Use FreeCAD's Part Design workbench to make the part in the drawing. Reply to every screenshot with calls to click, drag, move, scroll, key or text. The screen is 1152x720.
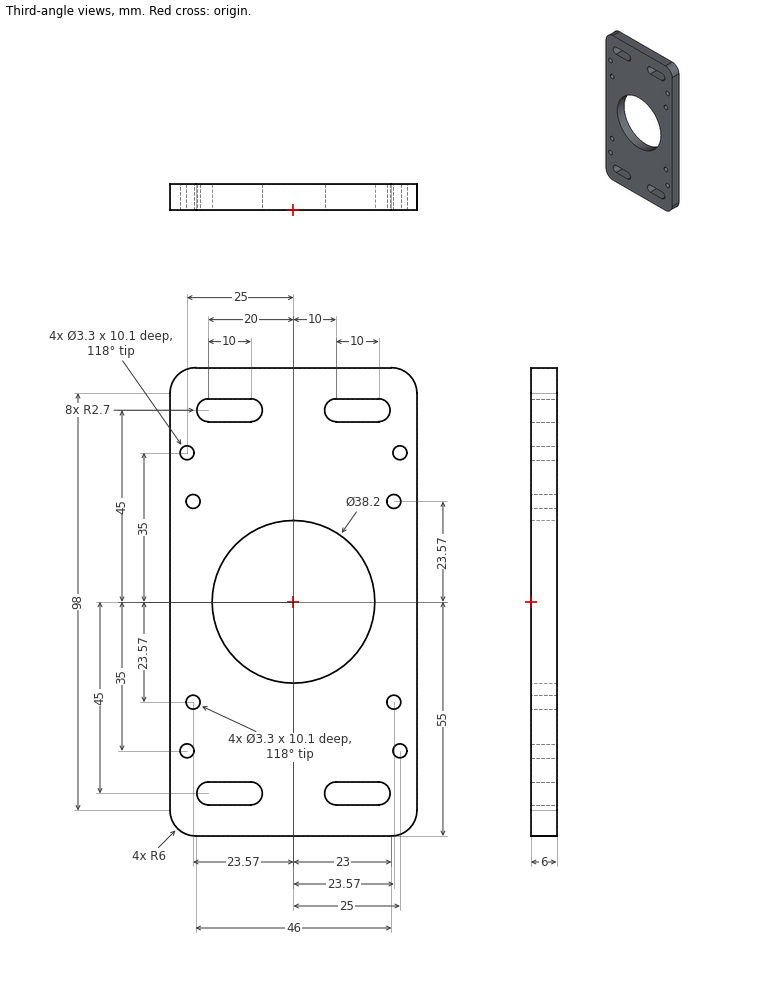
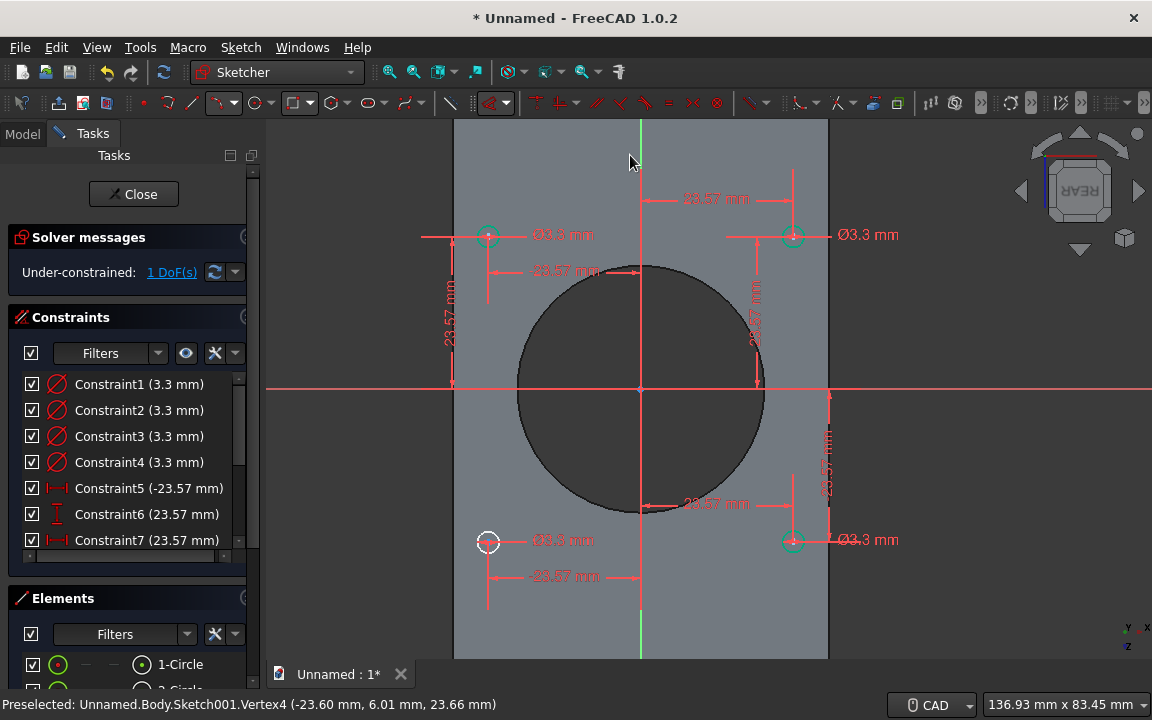
click(488, 542)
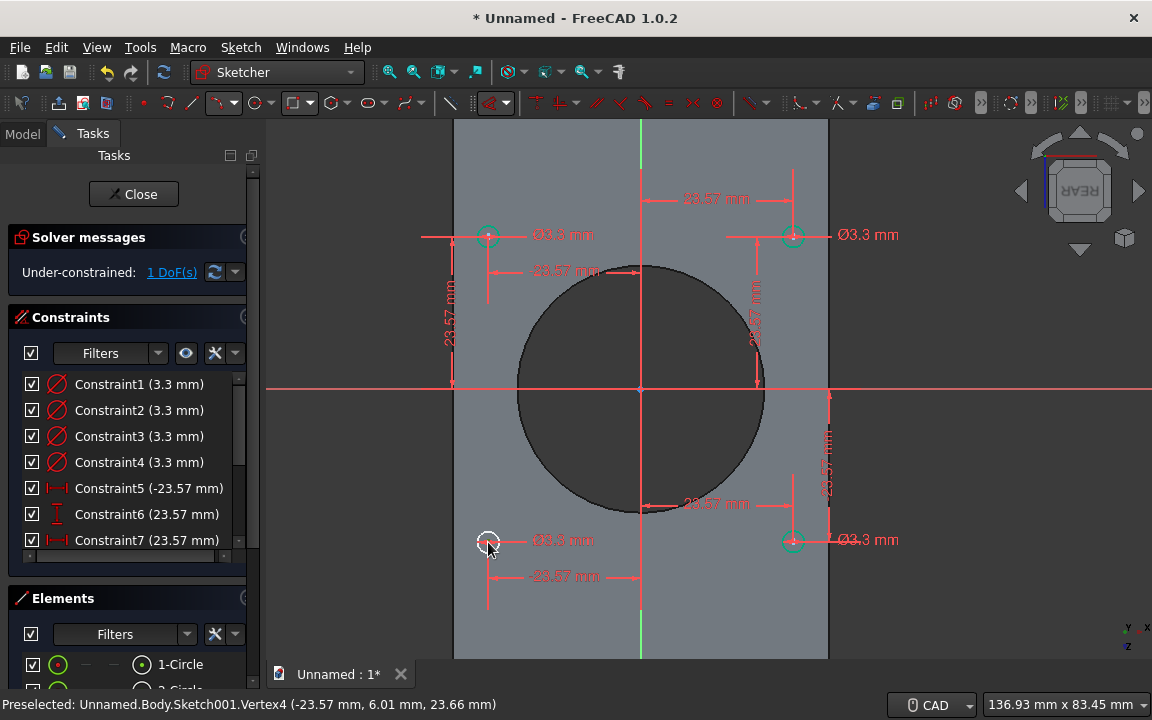
key(i)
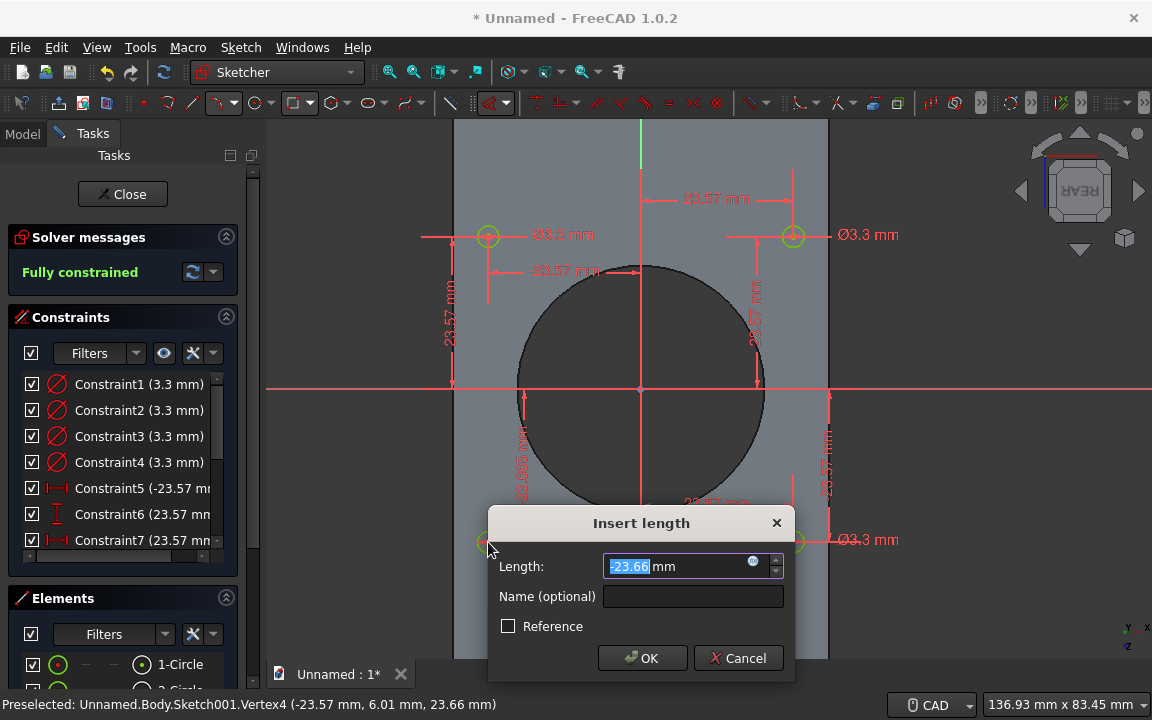
text(-23.57)
key(Return)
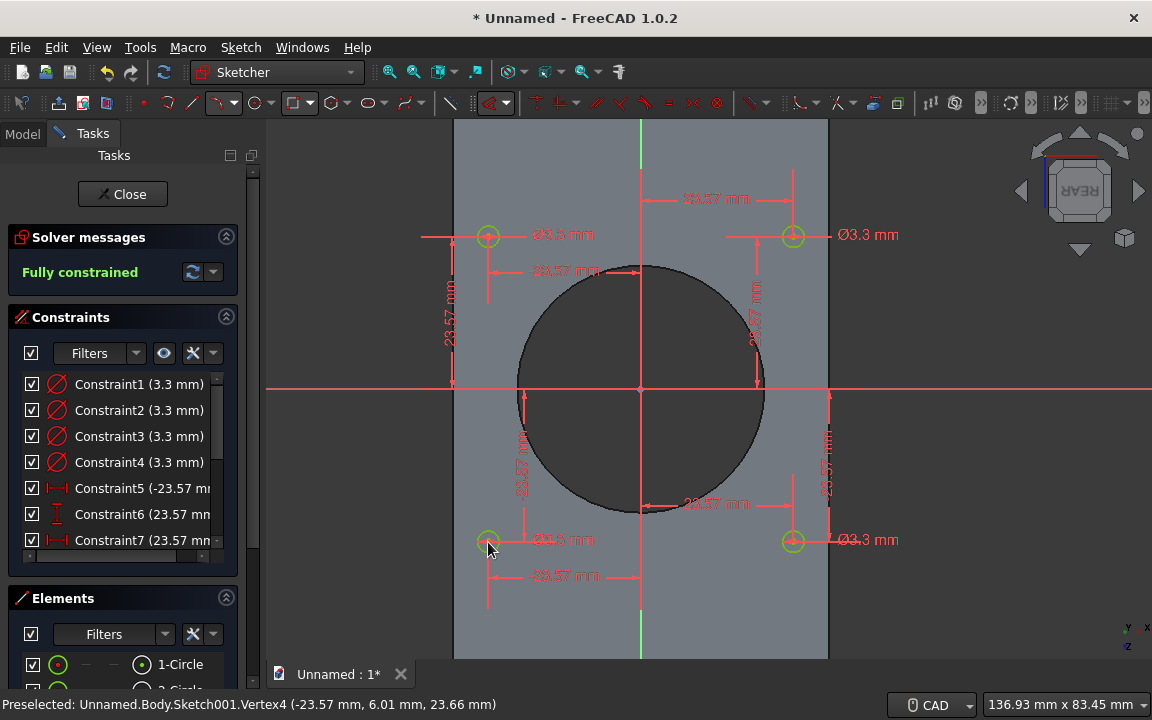
click(123, 194)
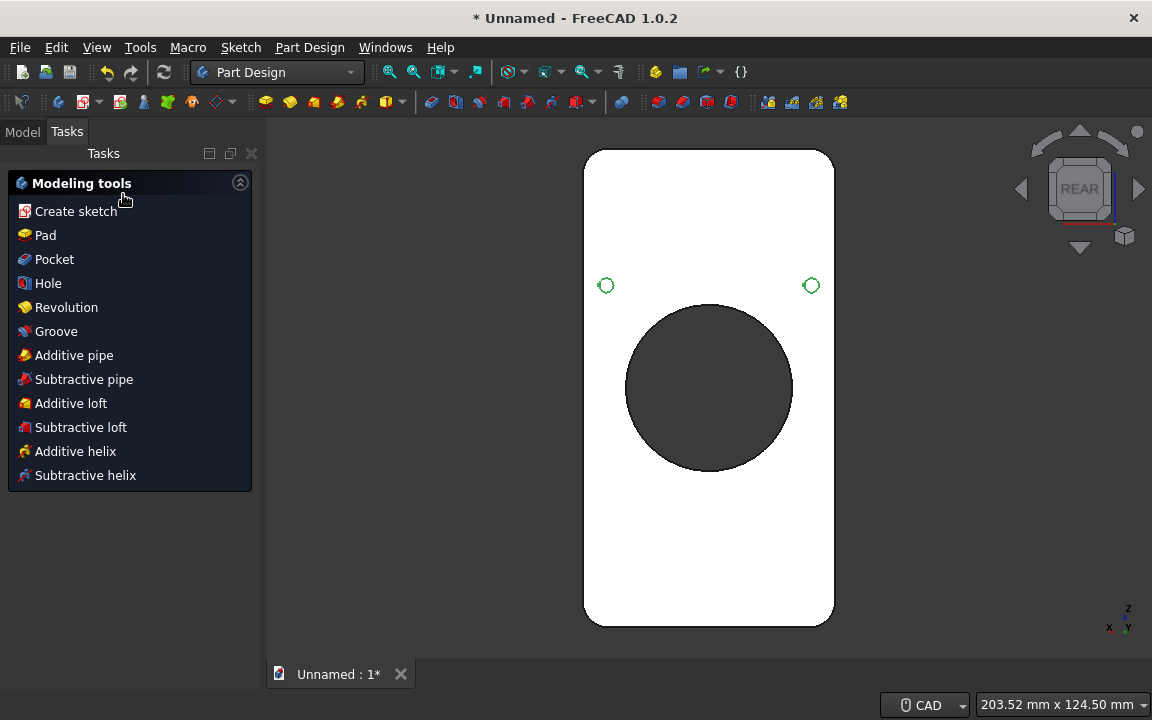
click(456, 102)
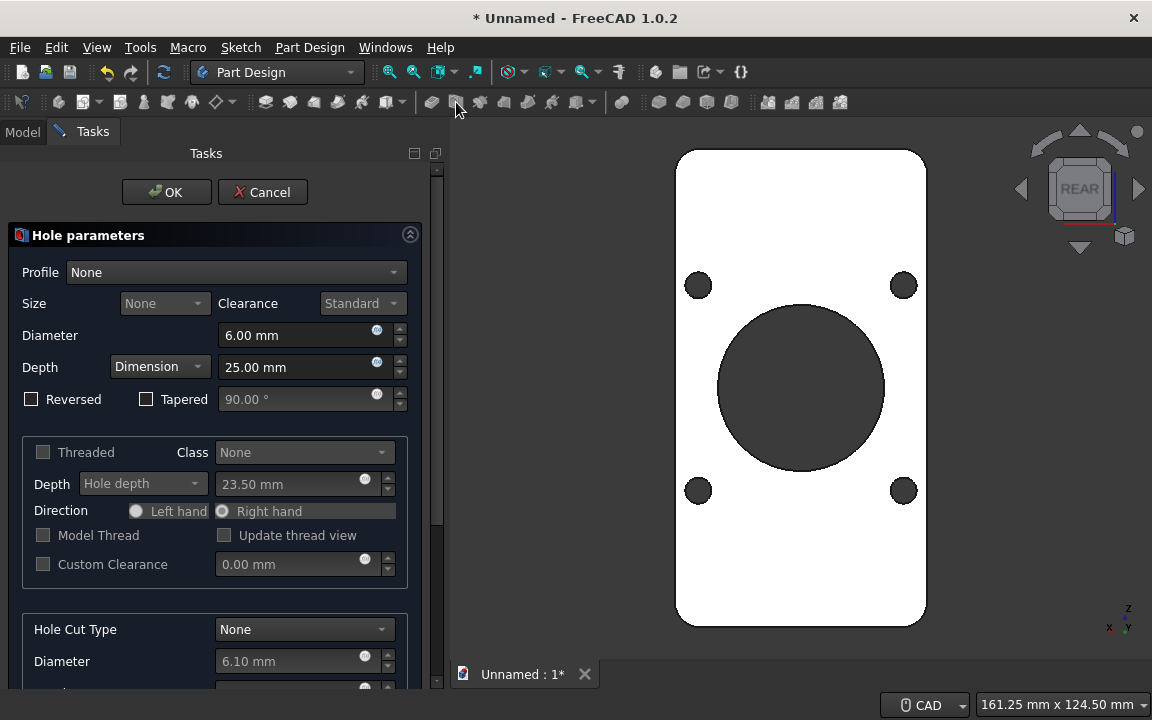
triple_click(305, 335)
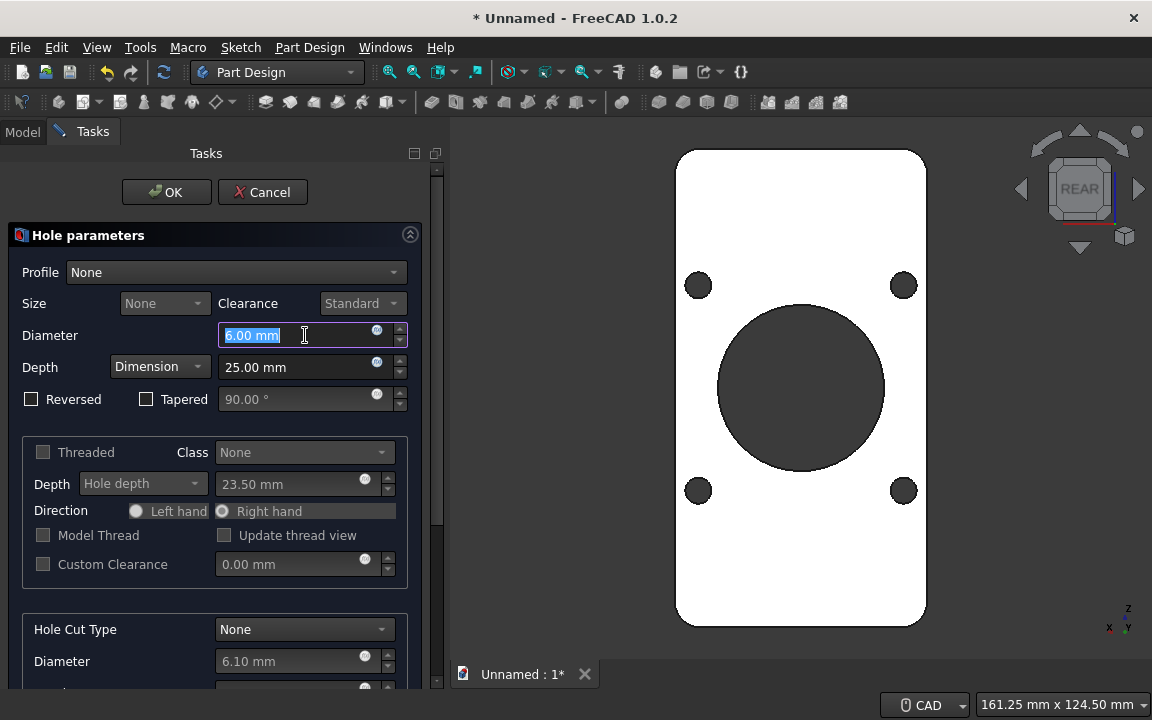
text(3.3)
key(Tab)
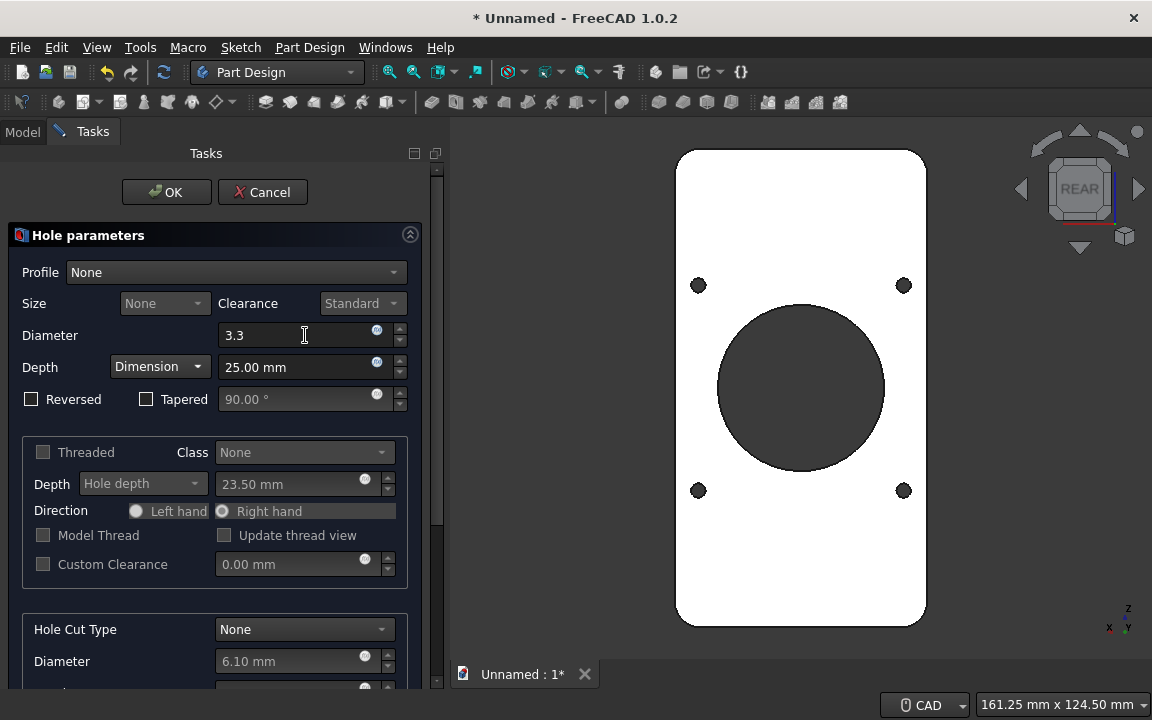
triple_click(305, 367)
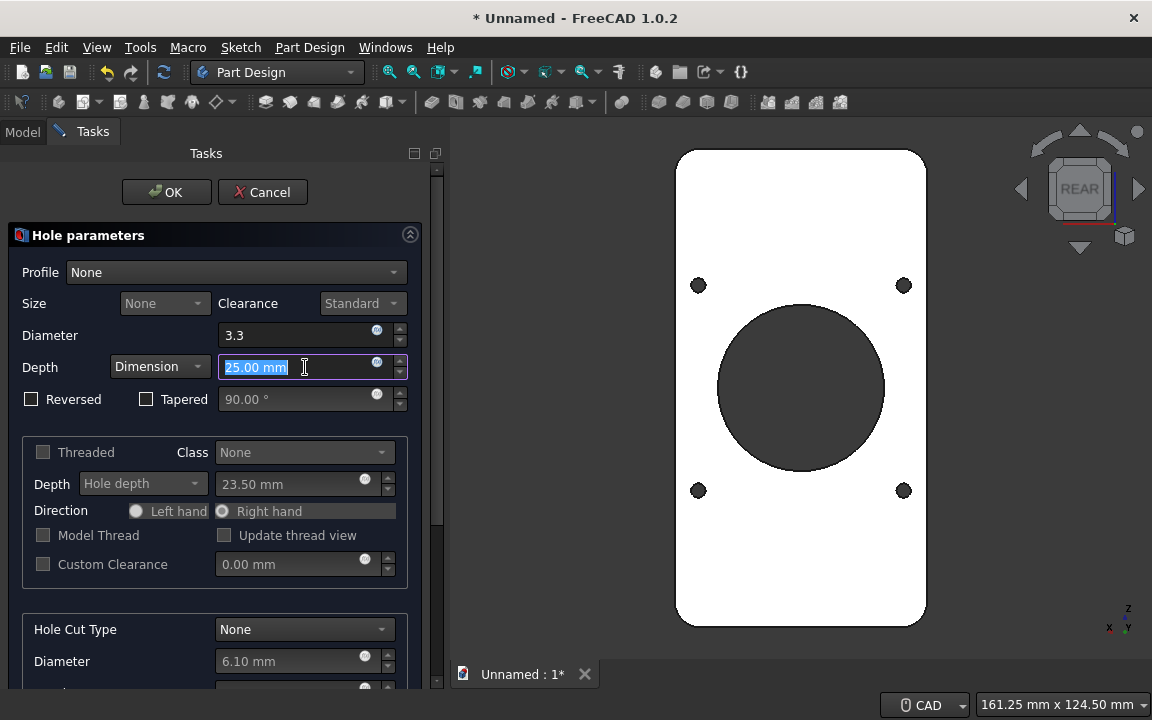
text(10.1)
key(Tab)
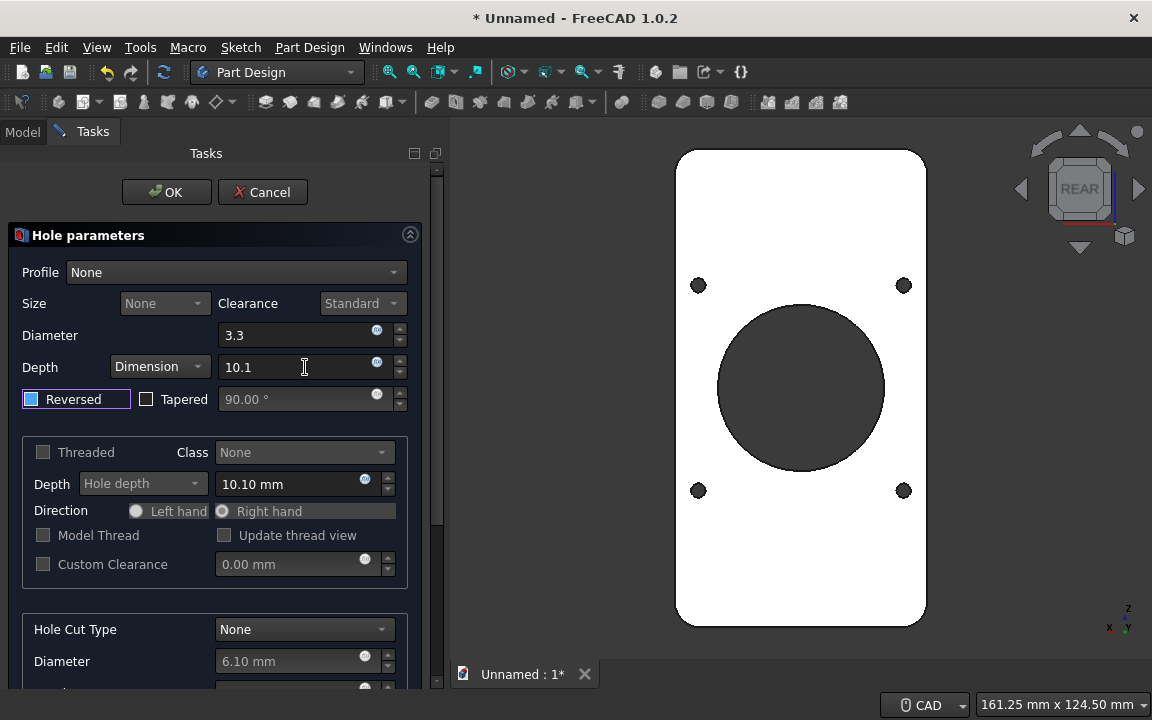
click(167, 192)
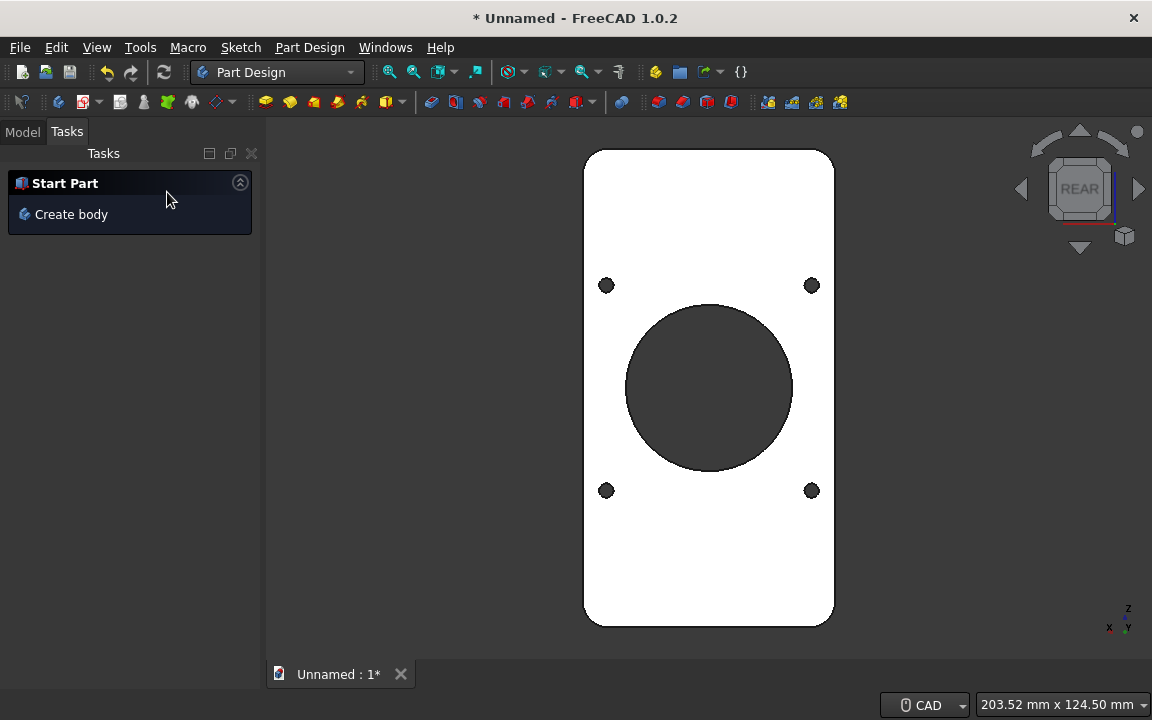
click(84, 102)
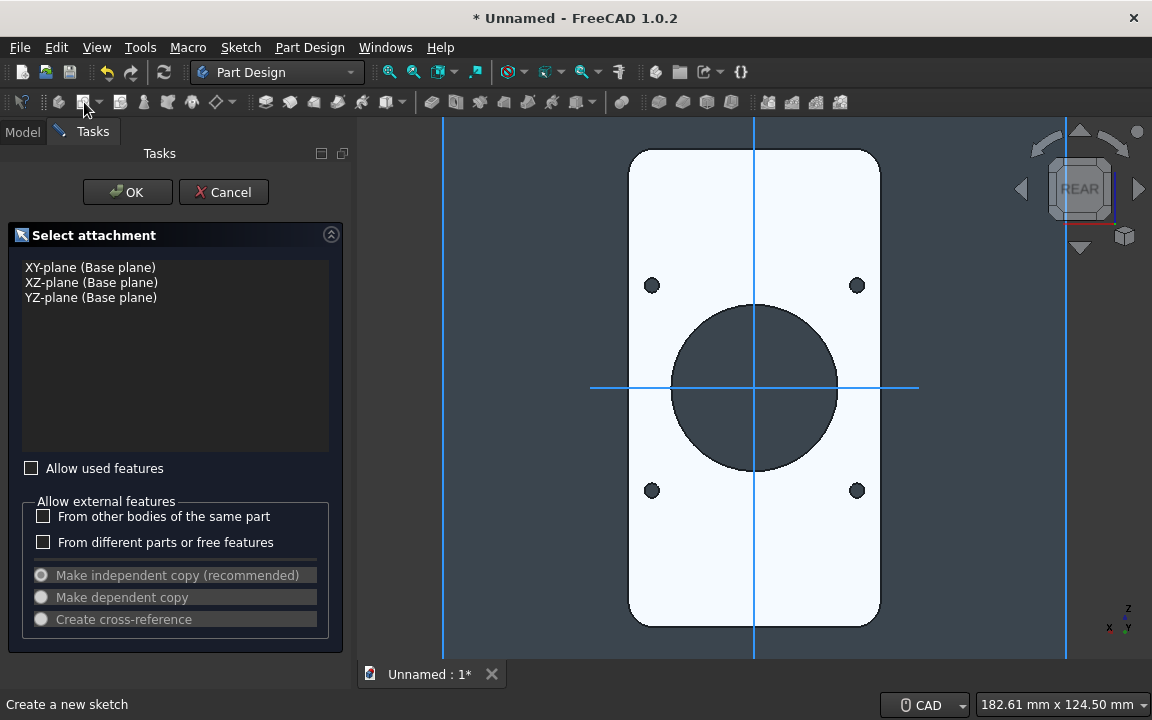
click(82, 282)